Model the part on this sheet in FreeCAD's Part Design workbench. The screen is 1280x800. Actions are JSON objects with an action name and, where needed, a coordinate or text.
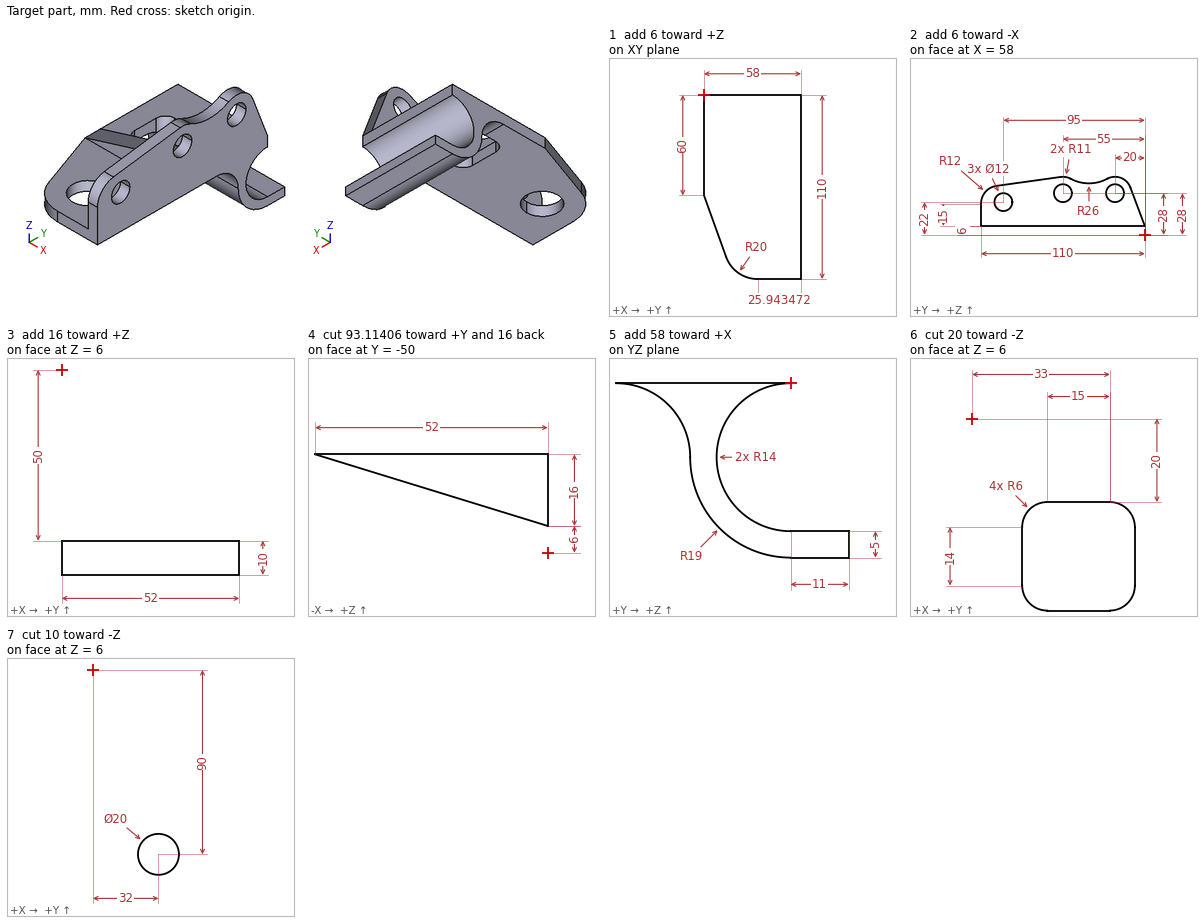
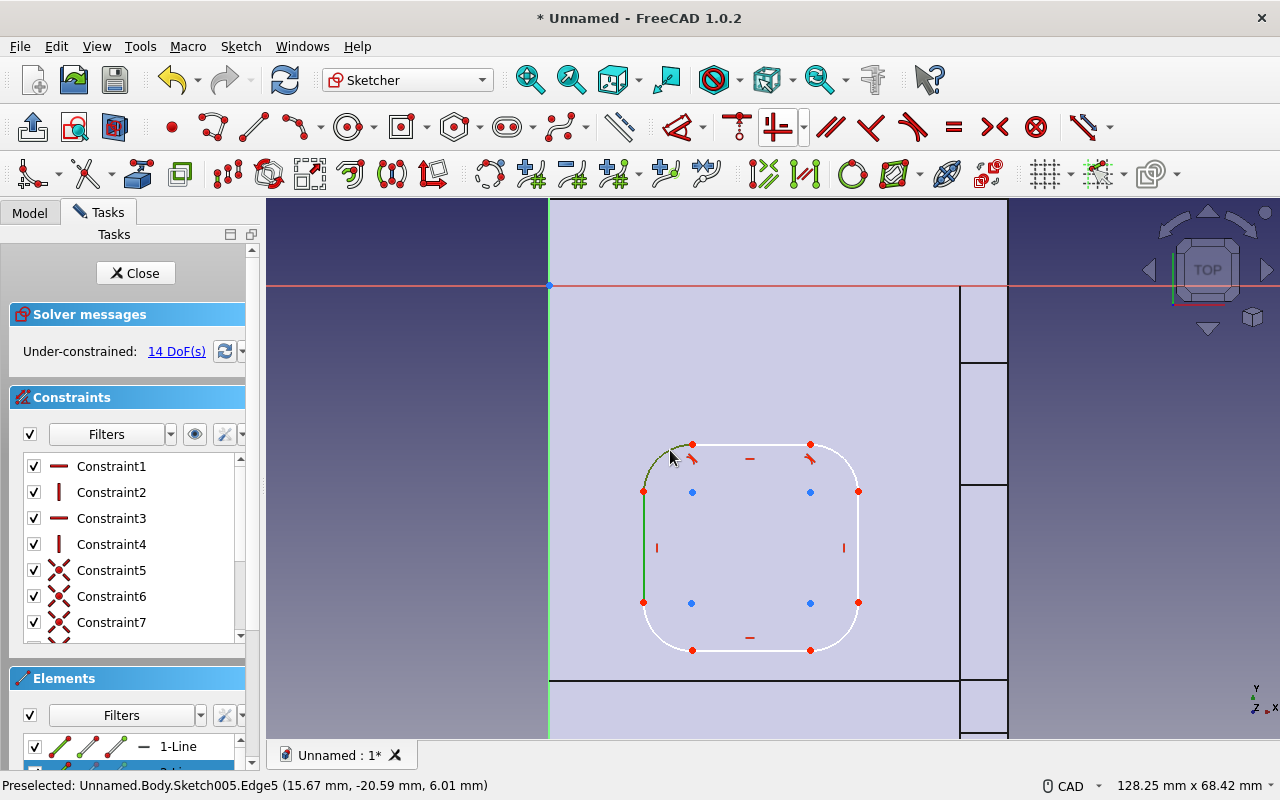
{"action": "left_click", "coordinate": [913, 128]}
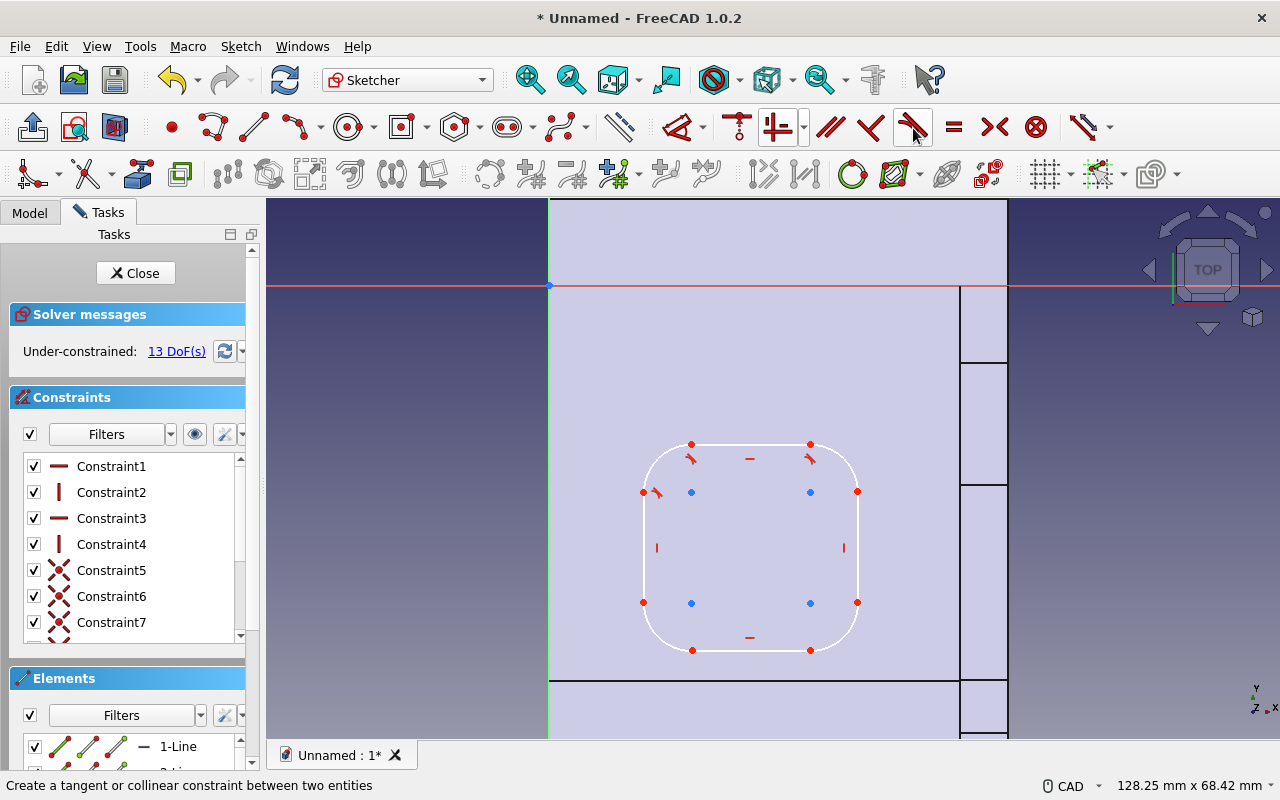
{"action": "left_click", "coordinate": [644, 526]}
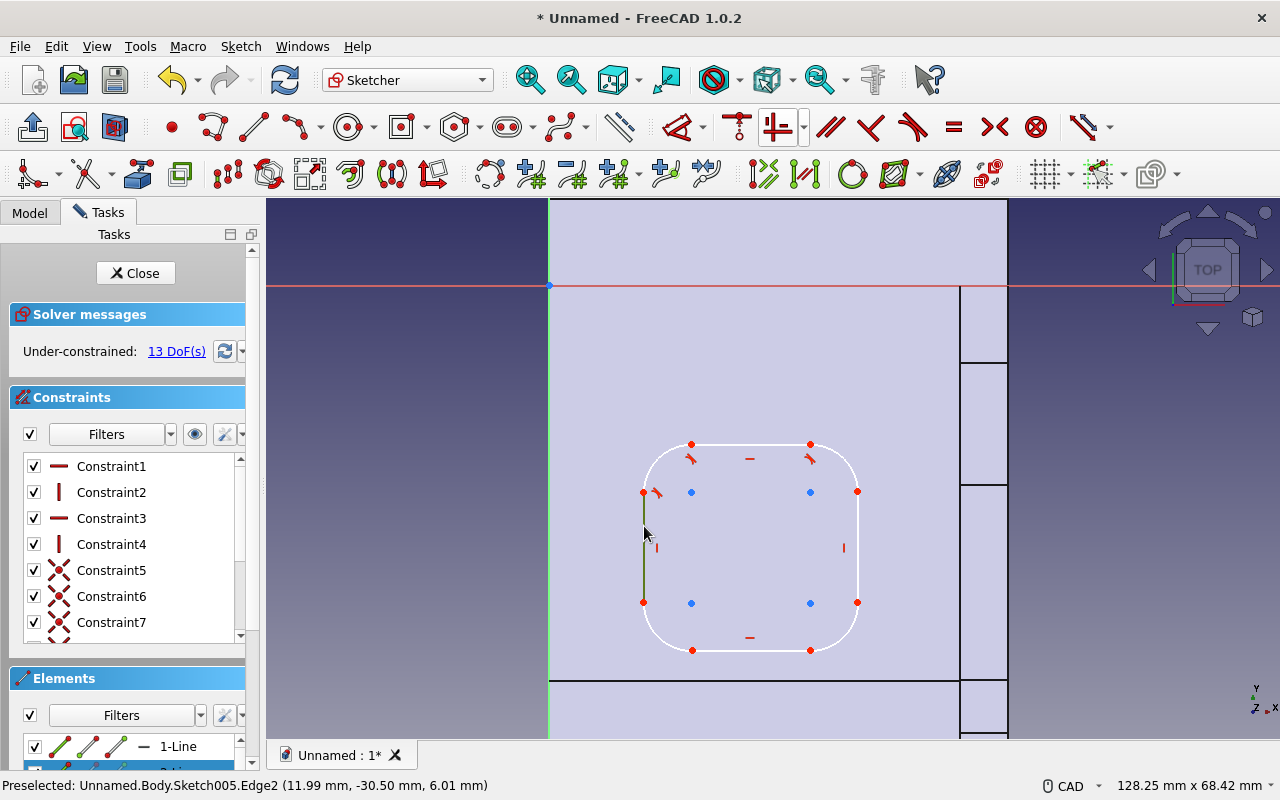
{"action": "left_click", "coordinate": [649, 625]}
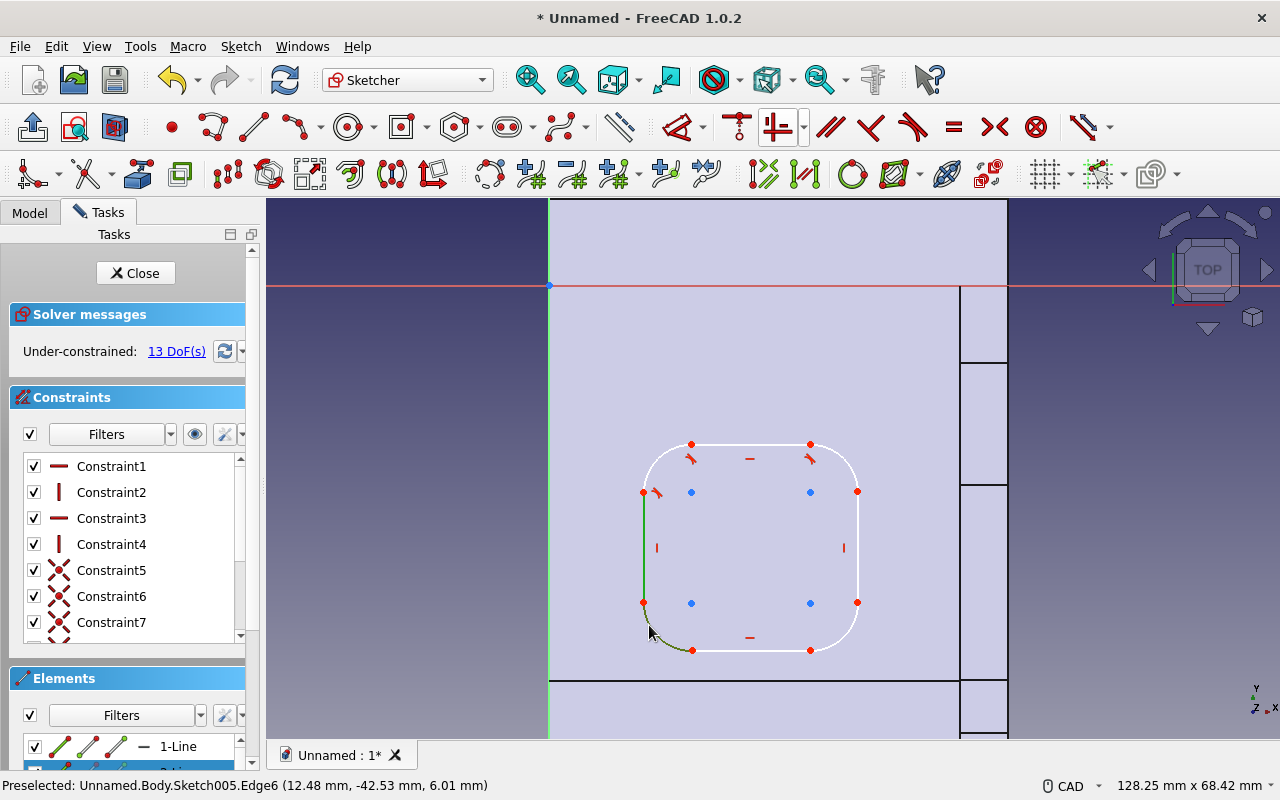
{"action": "key", "text": "t"}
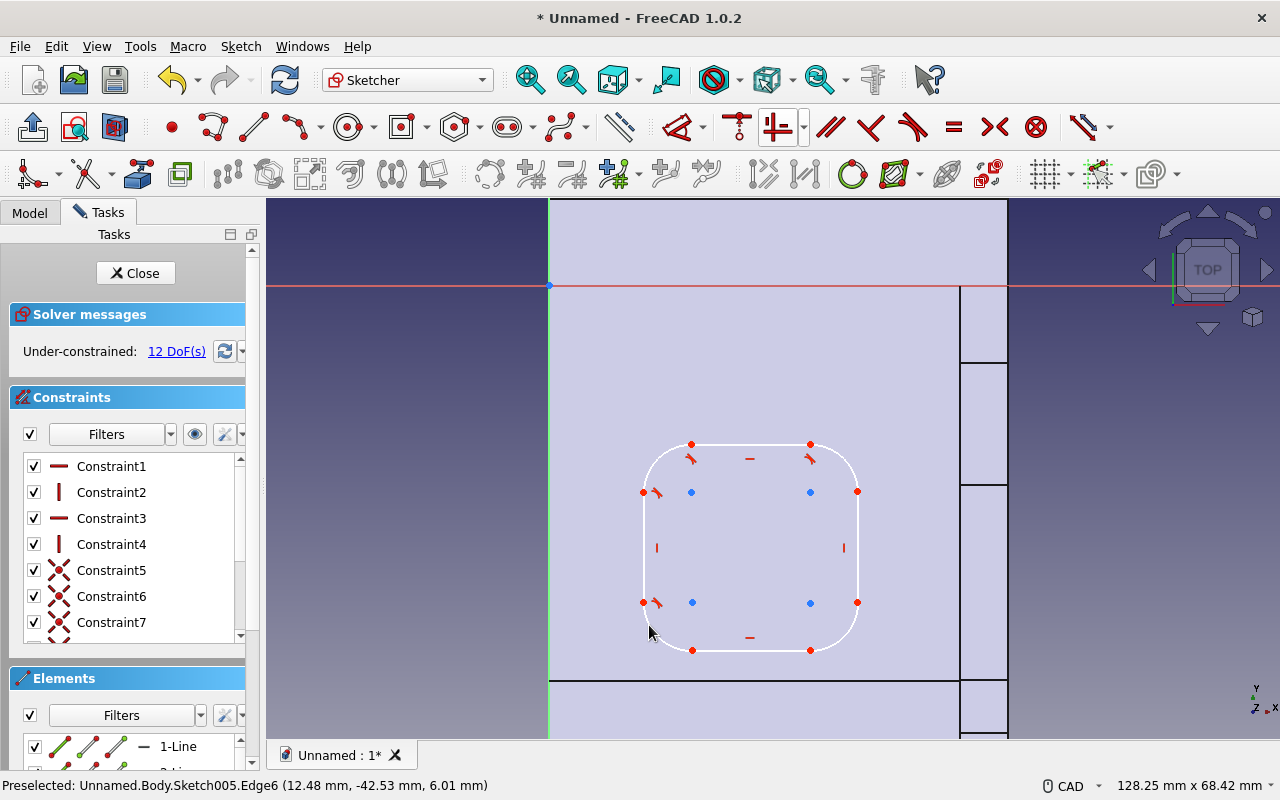
{"action": "left_click", "coordinate": [727, 651]}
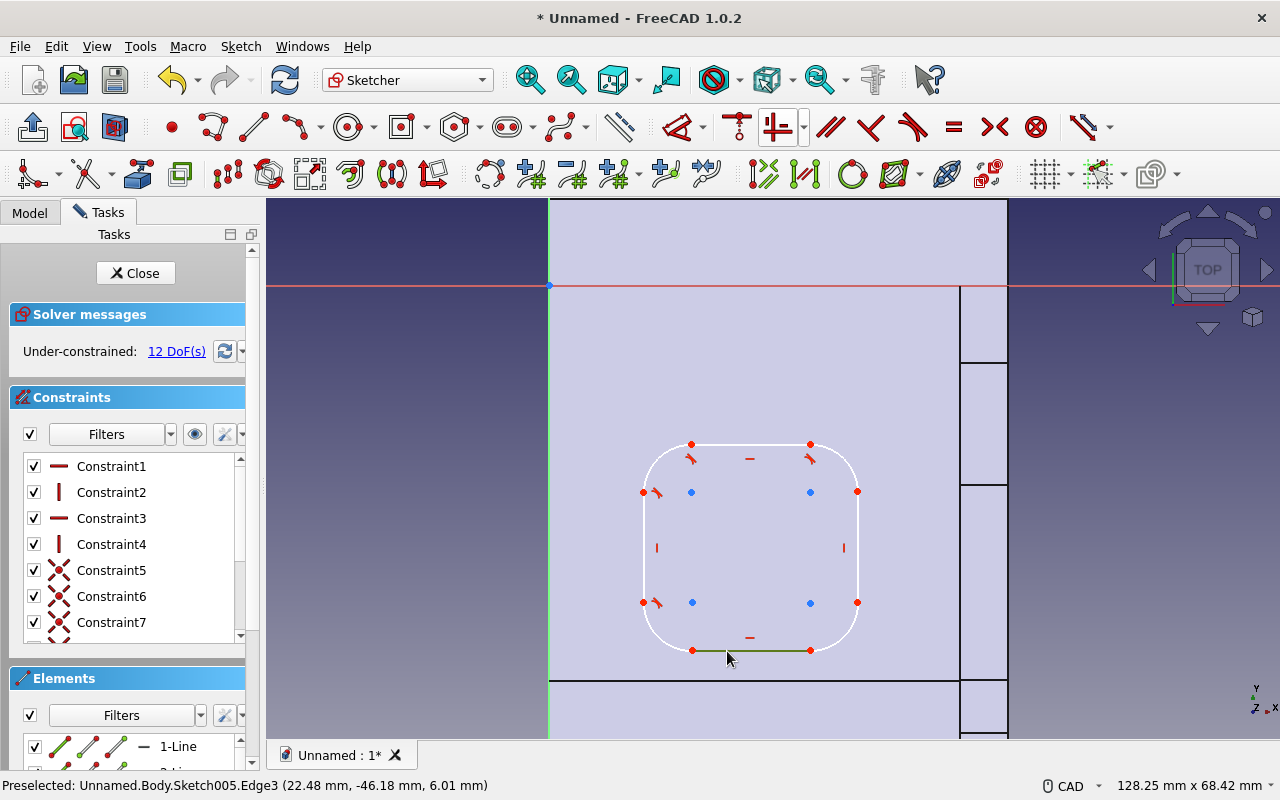
{"action": "left_click", "coordinate": [649, 625]}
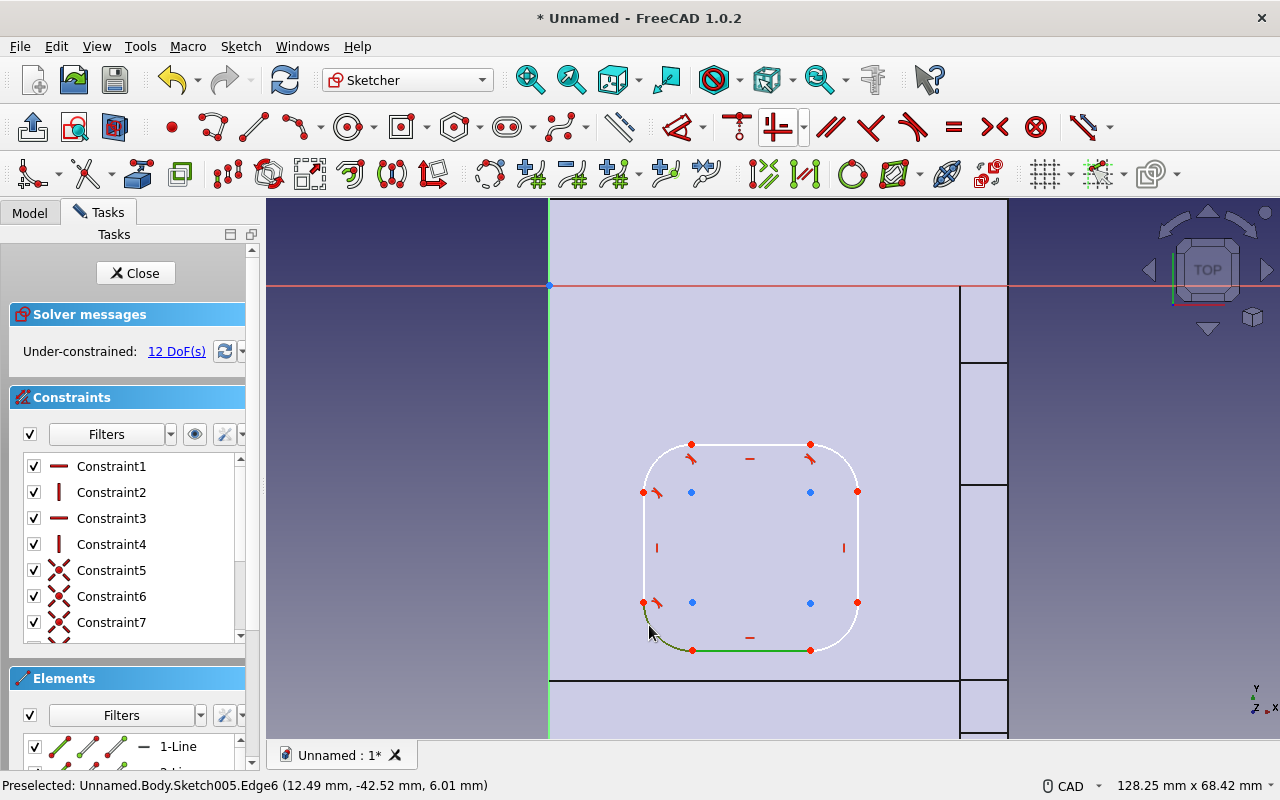
{"action": "left_click", "coordinate": [913, 128]}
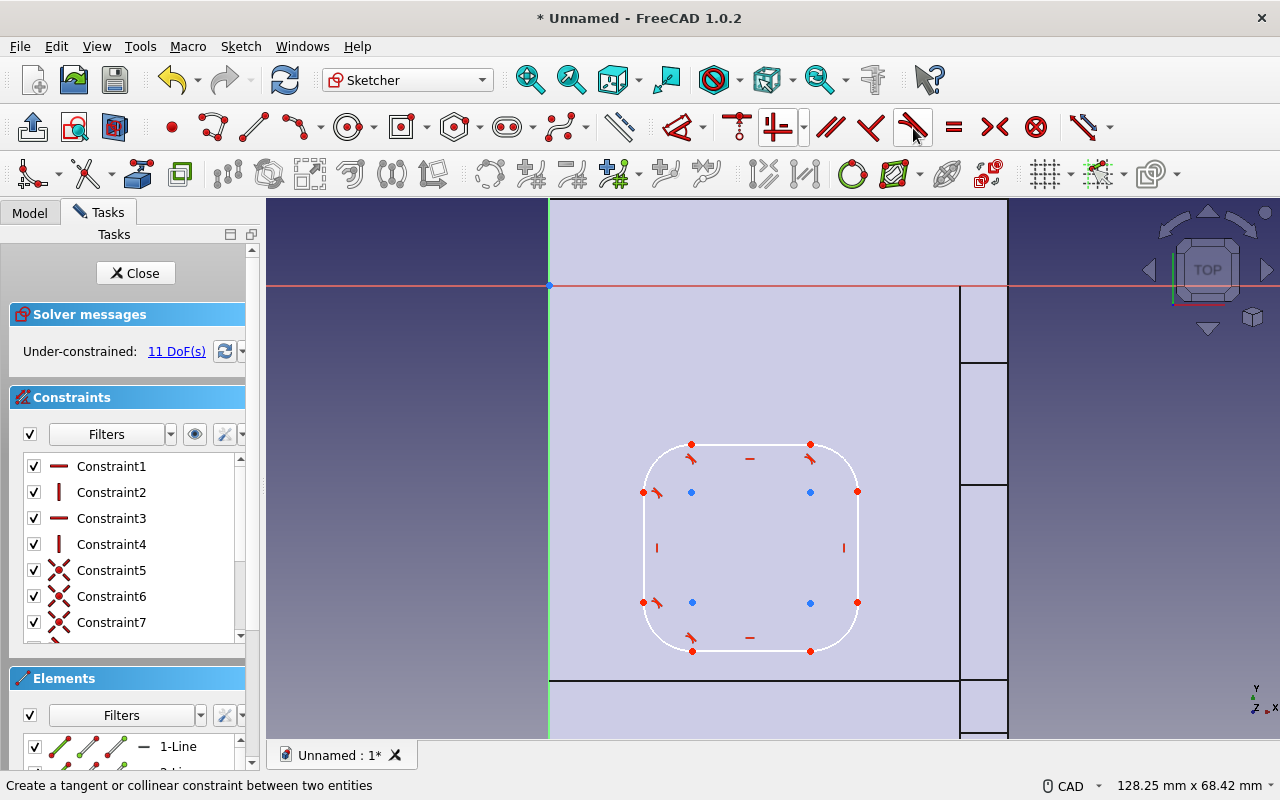
{"action": "left_click", "coordinate": [727, 651]}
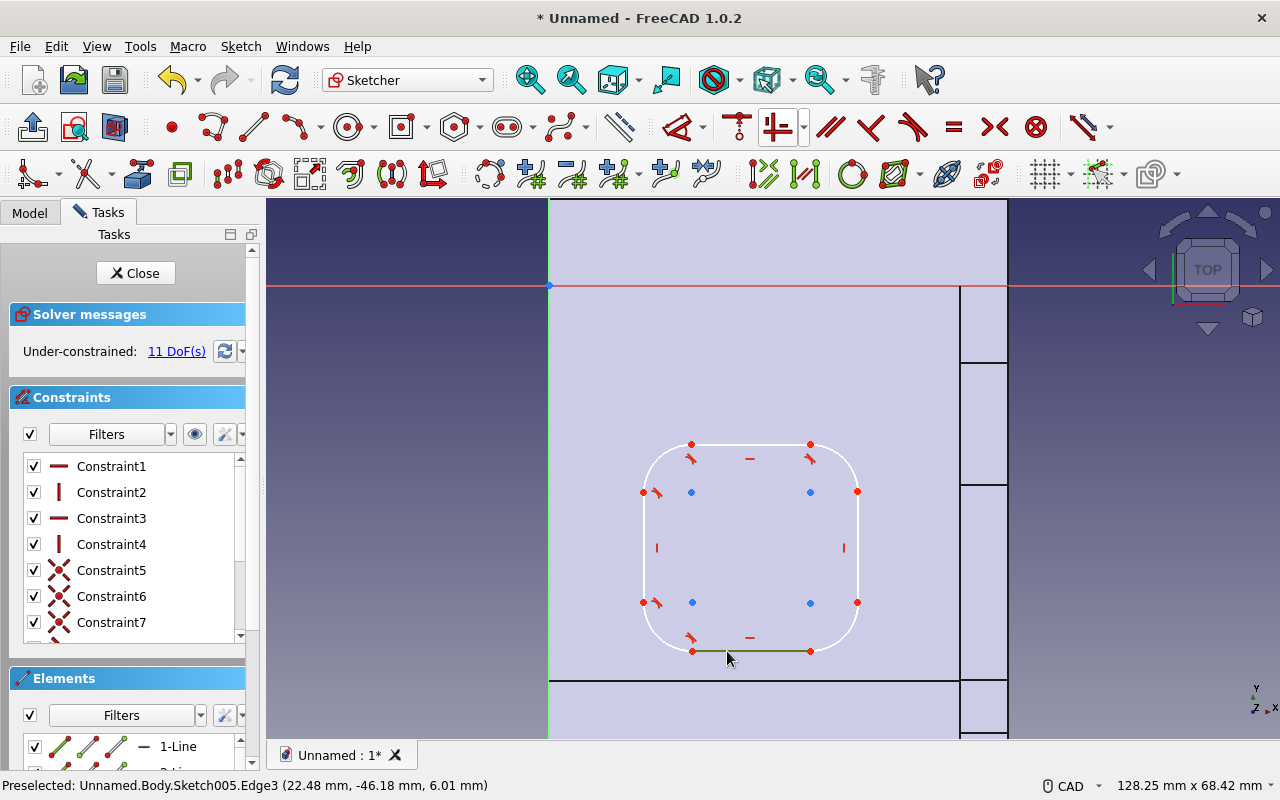
{"action": "left_click", "coordinate": [832, 646]}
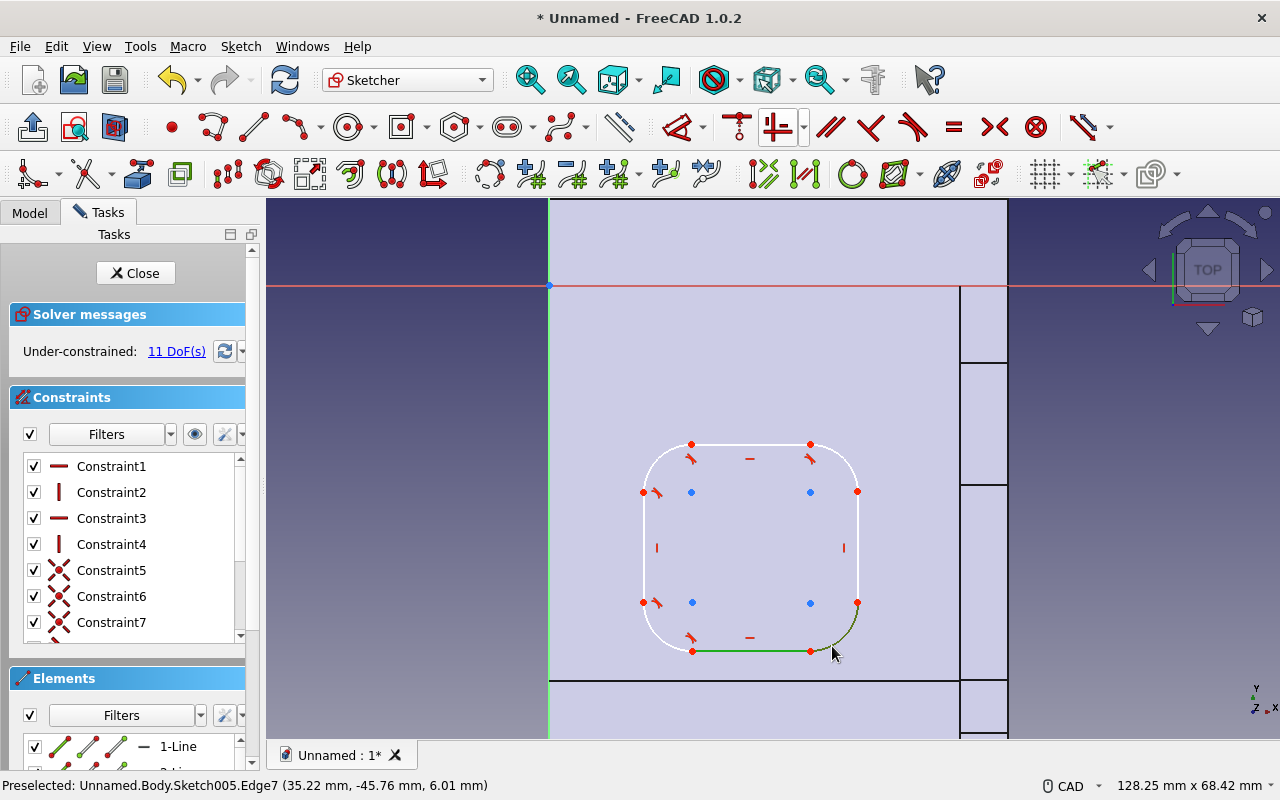
{"action": "left_click", "coordinate": [913, 128]}